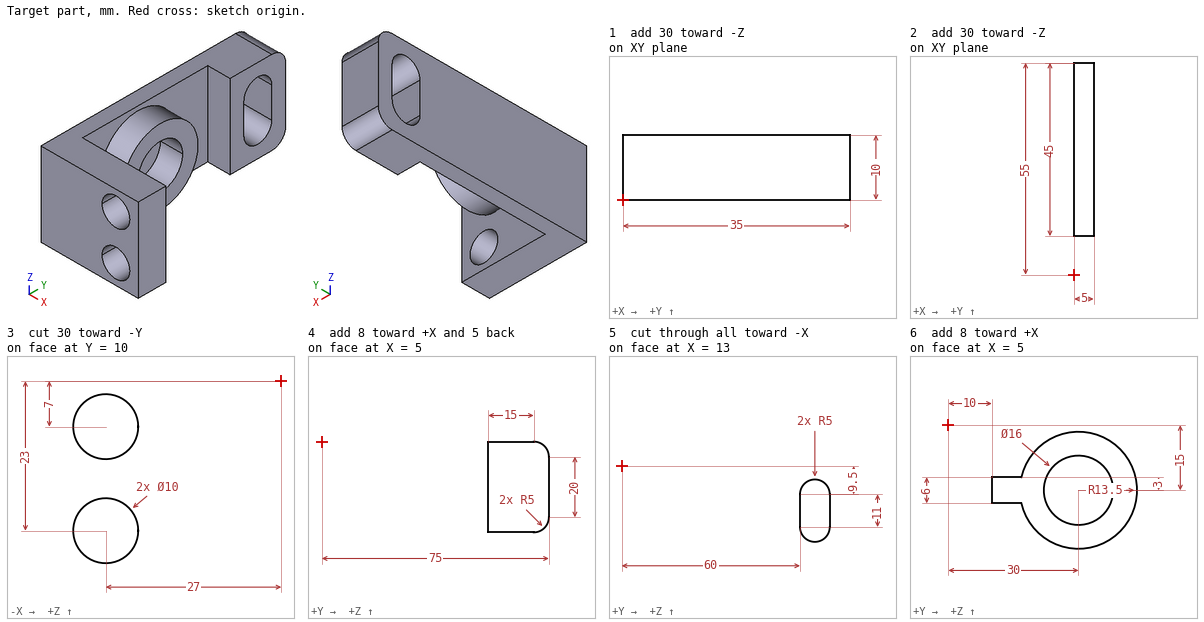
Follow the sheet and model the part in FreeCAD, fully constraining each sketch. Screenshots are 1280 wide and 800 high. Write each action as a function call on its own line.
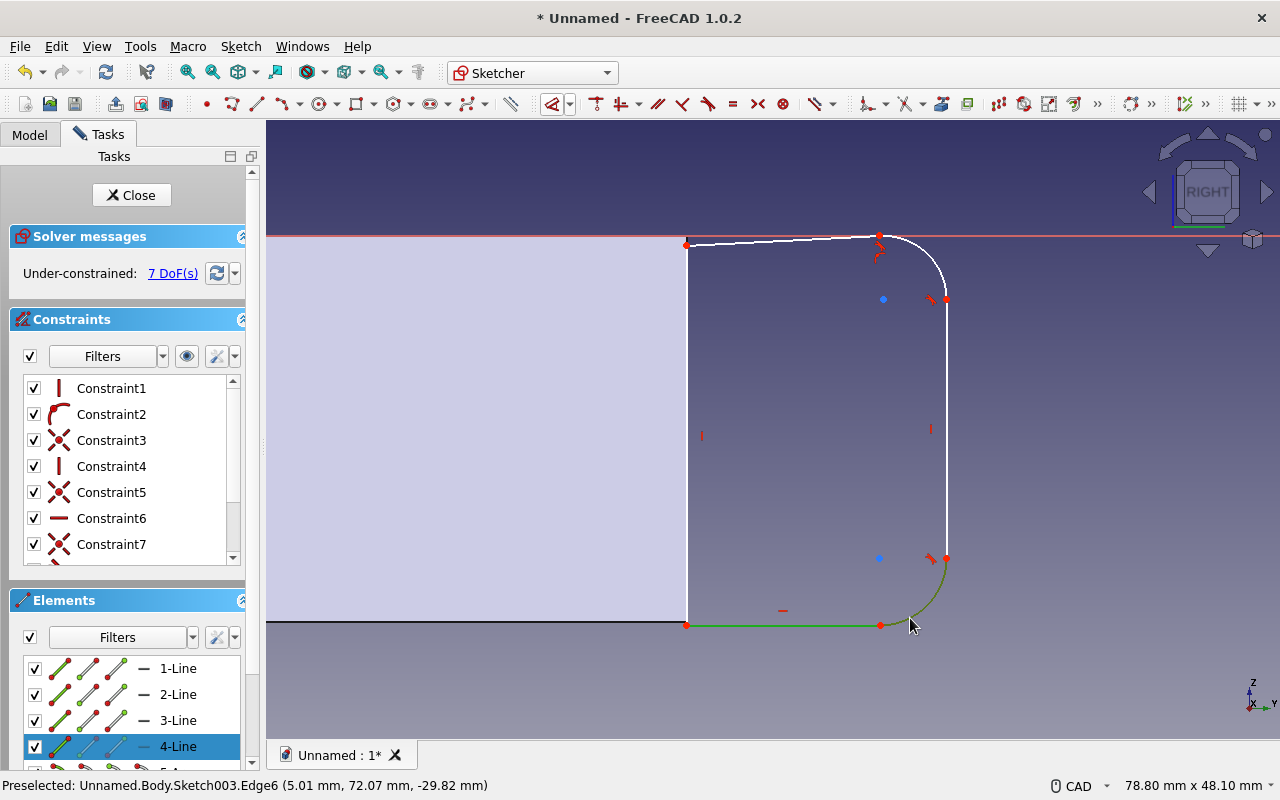
key(t)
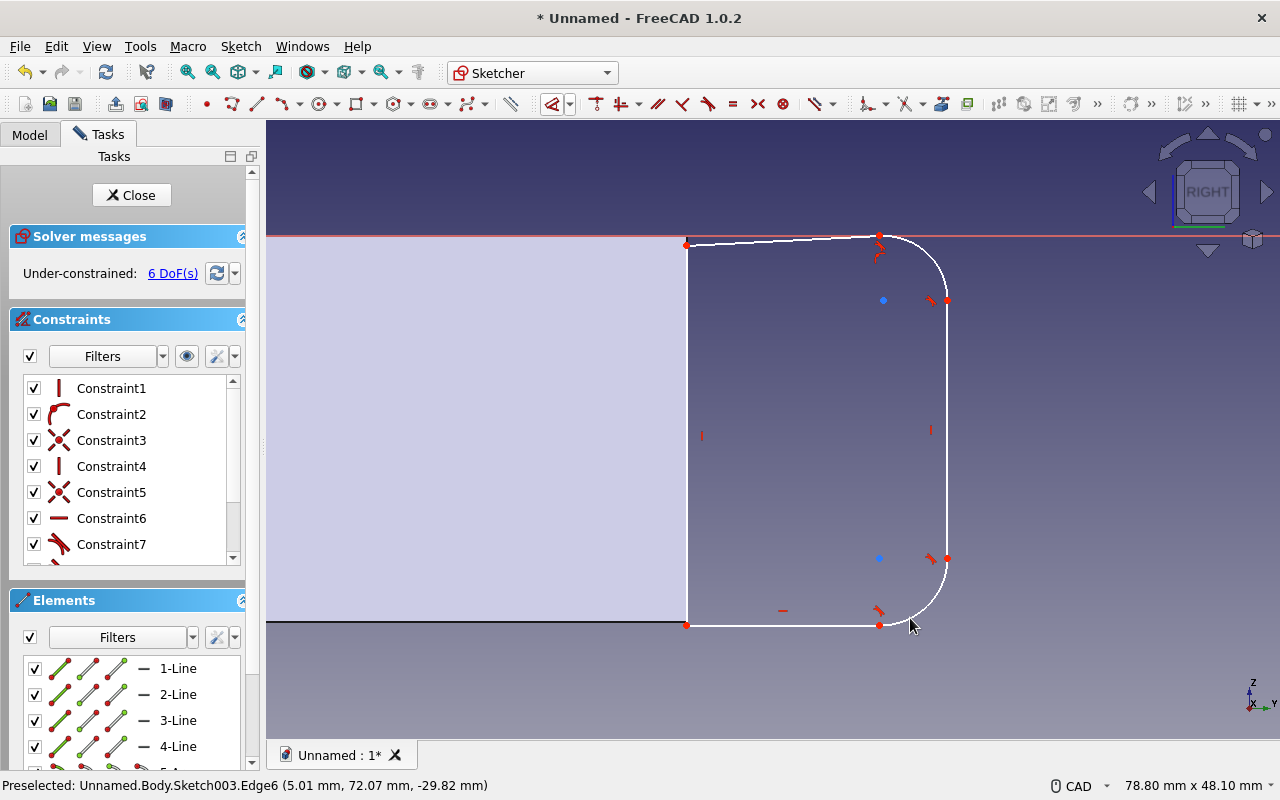
click(822, 239)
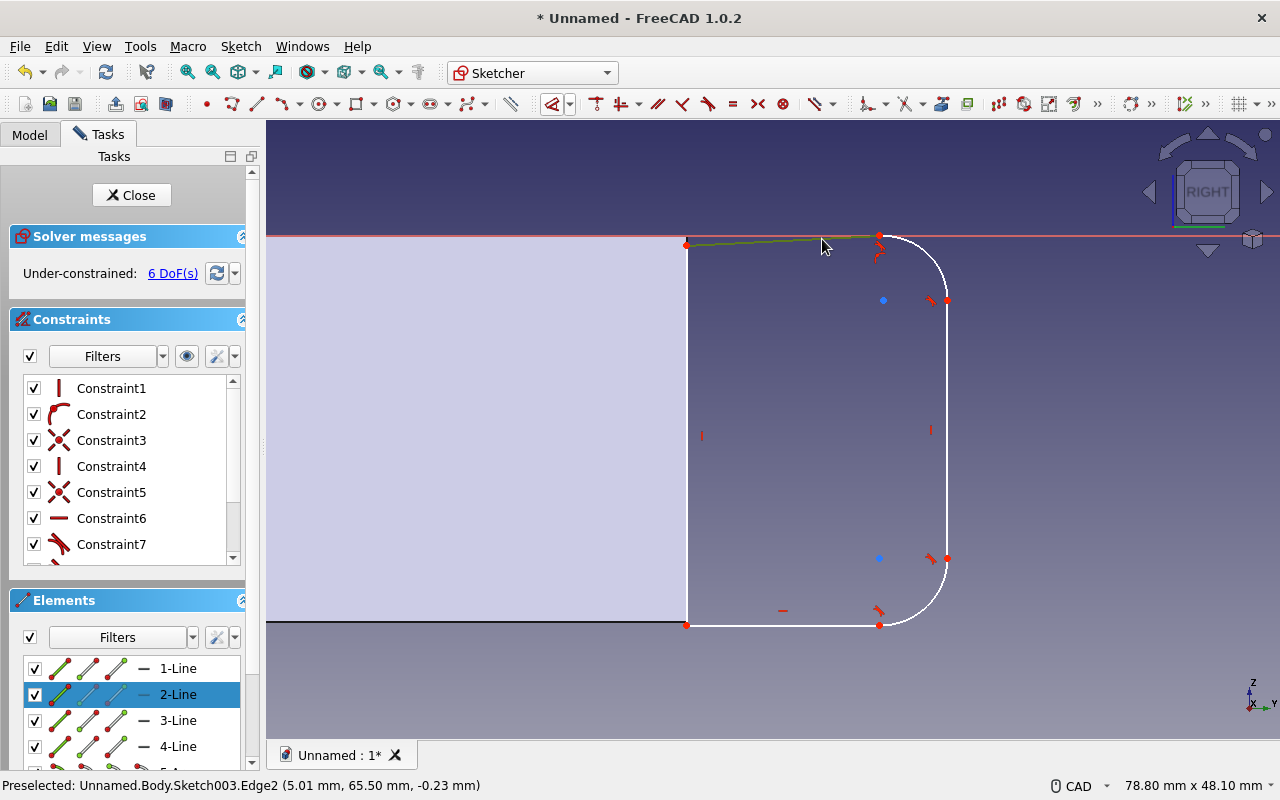
key(h)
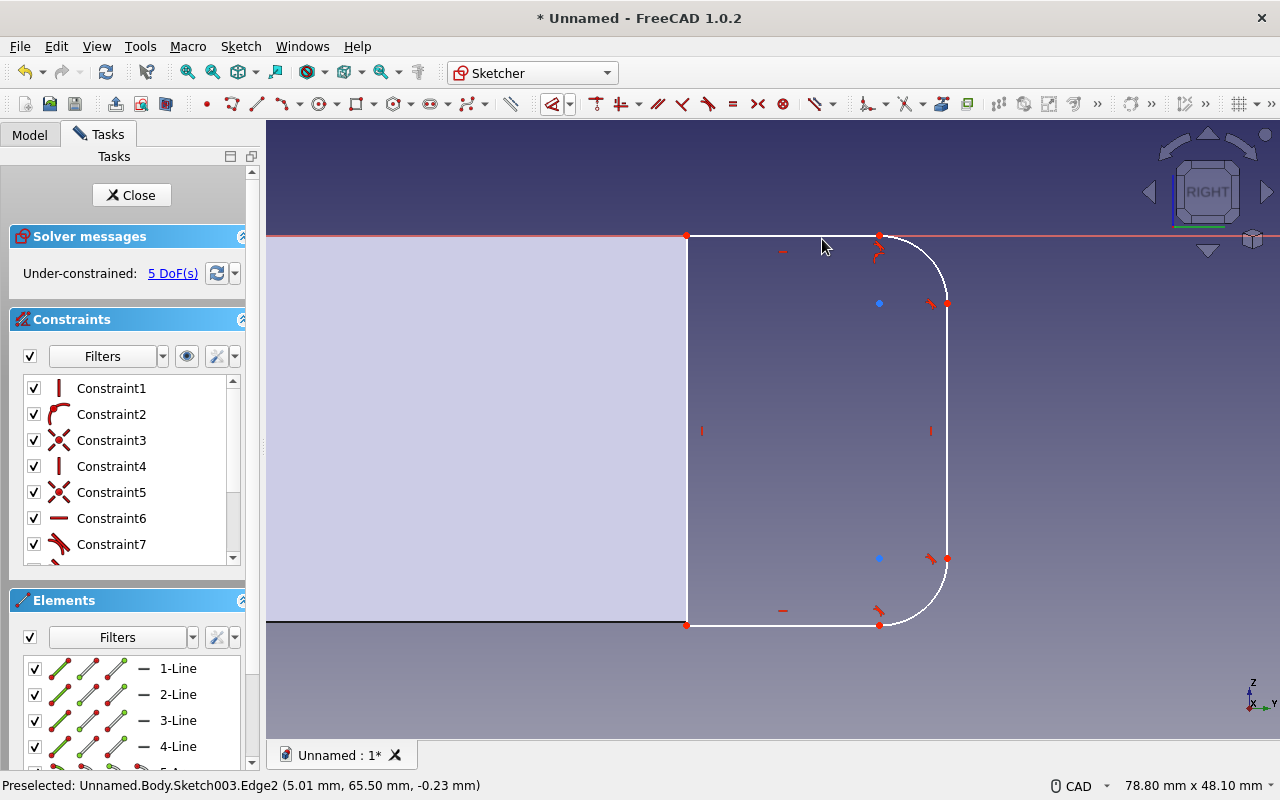
click(940, 273)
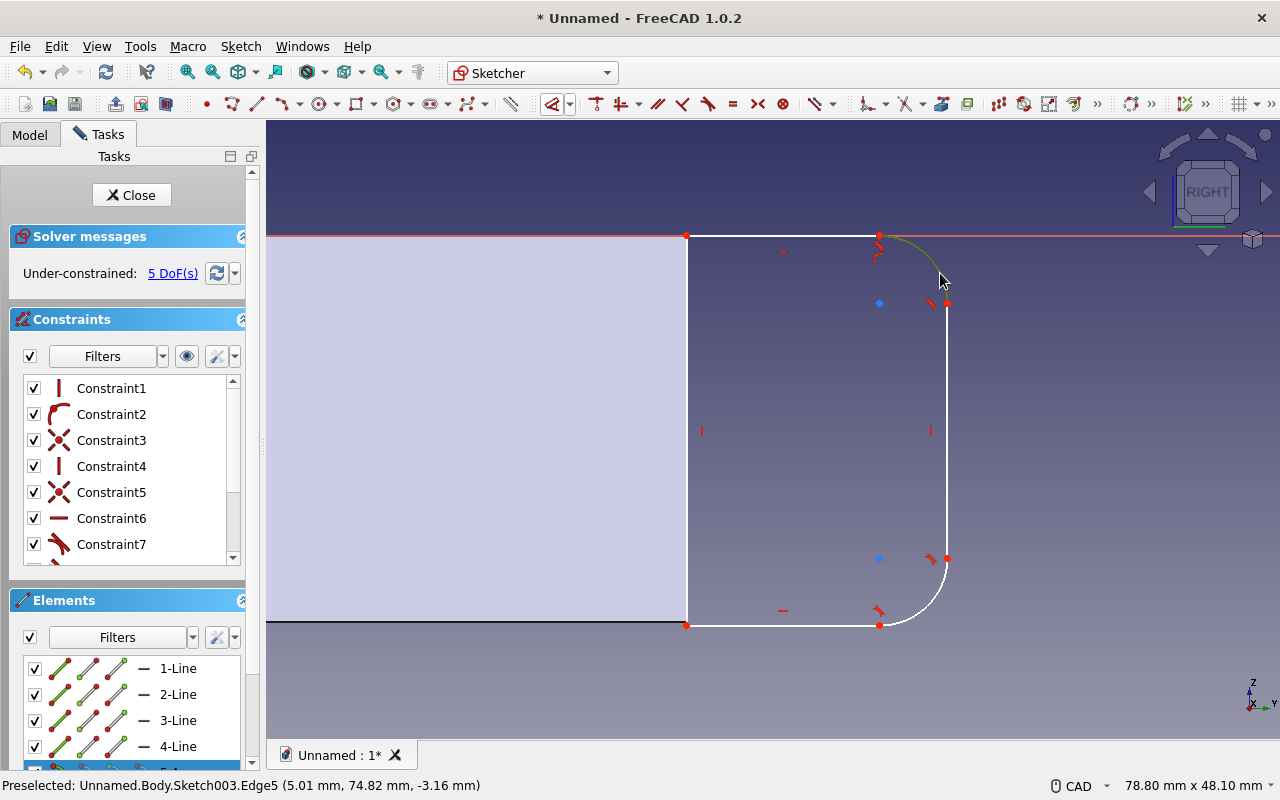
click(911, 618)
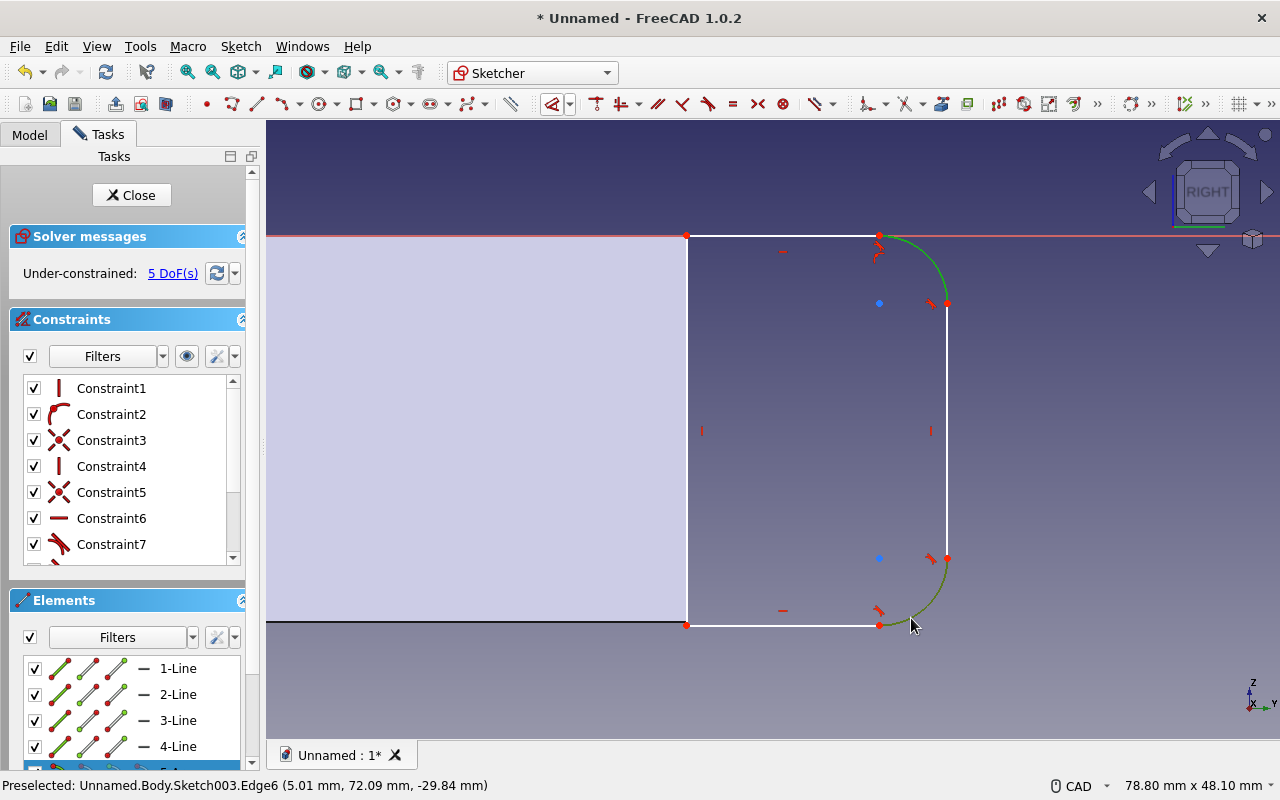
key(e)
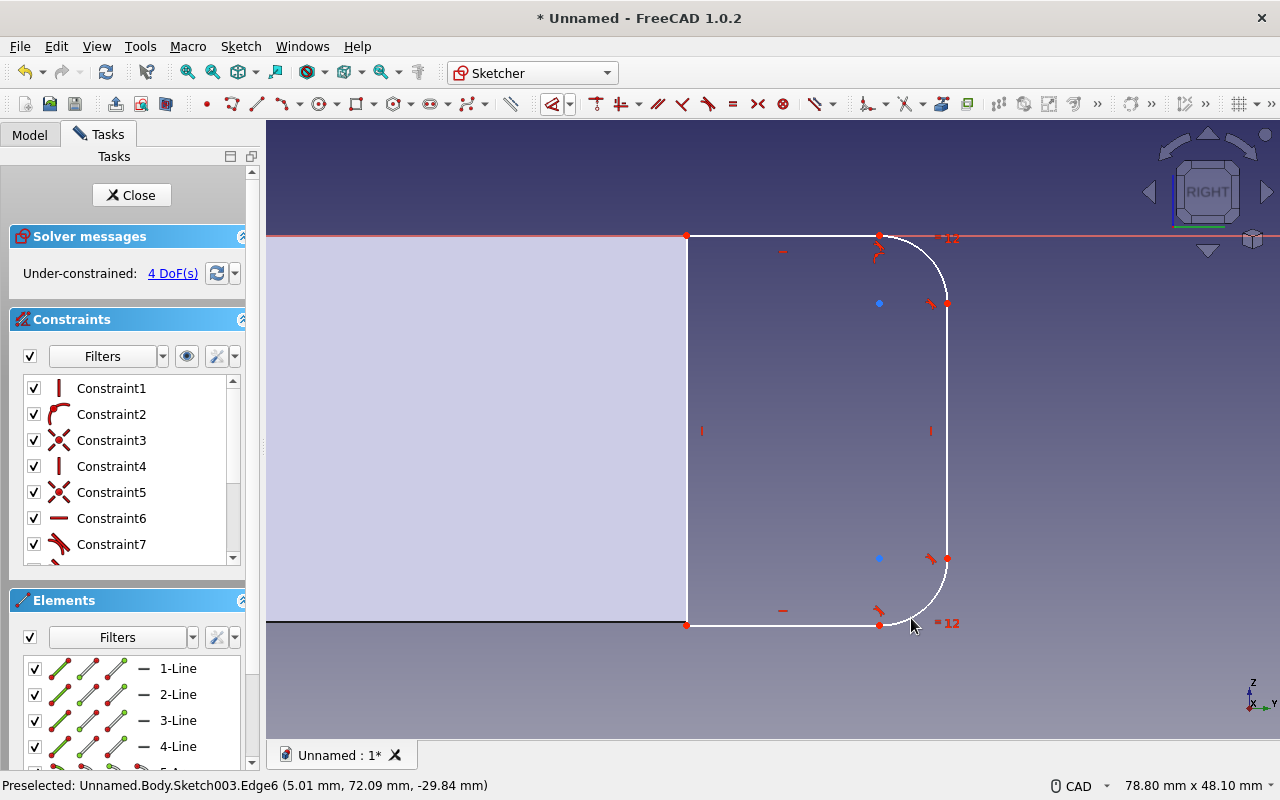
key(d)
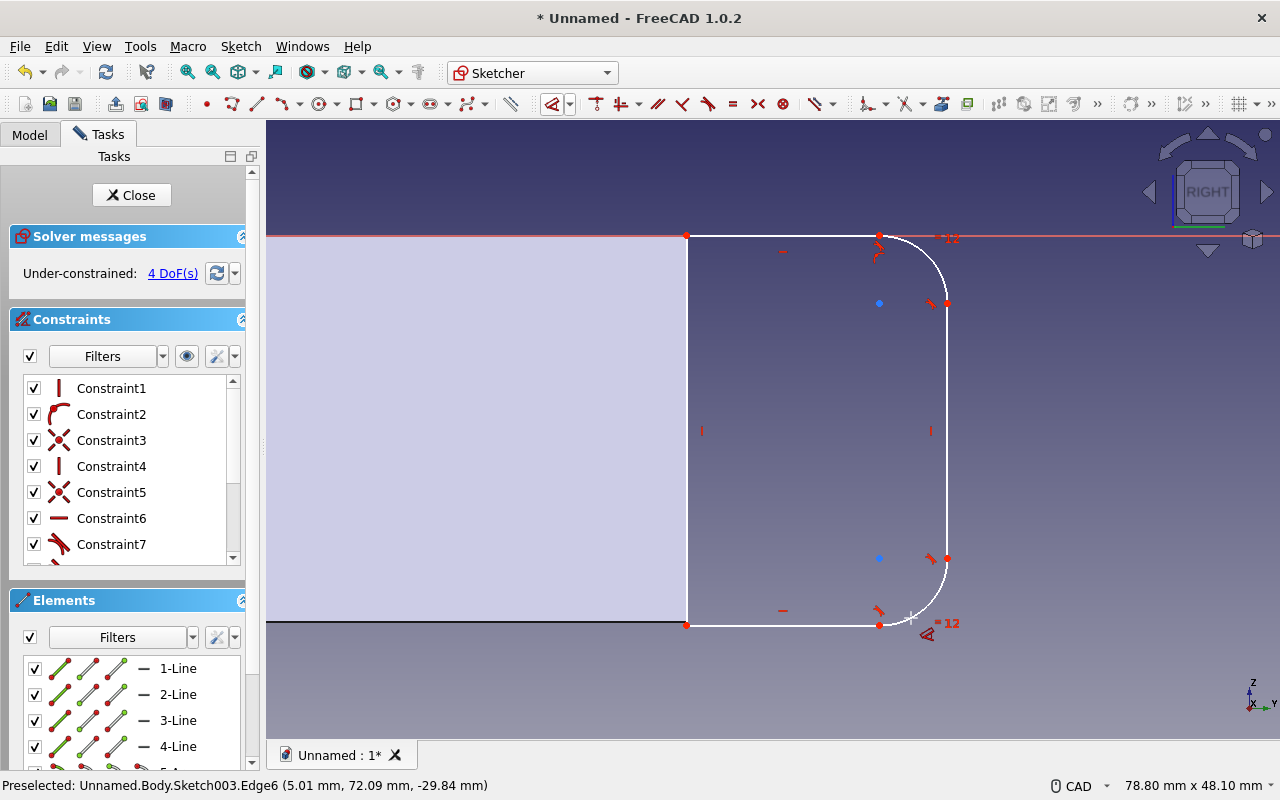
click(940, 273)
click(969, 259)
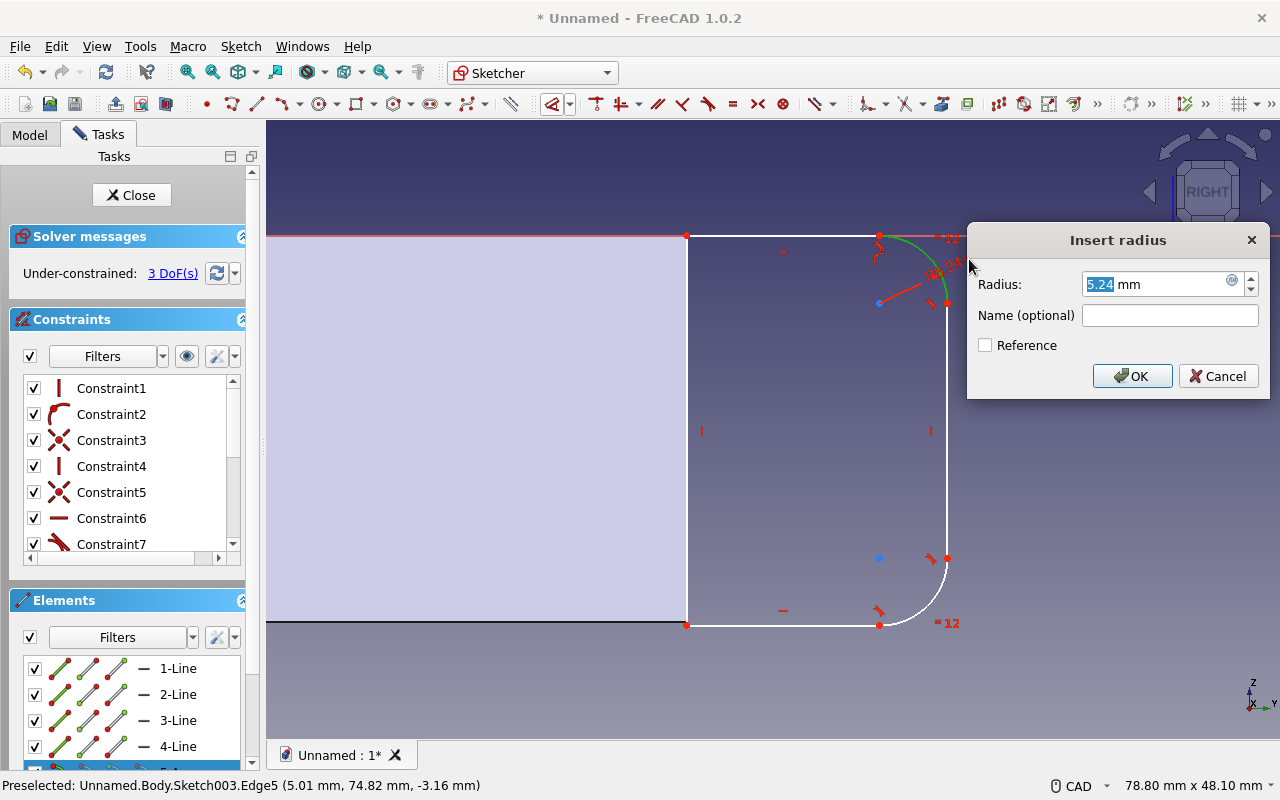
text(5)
key(Return)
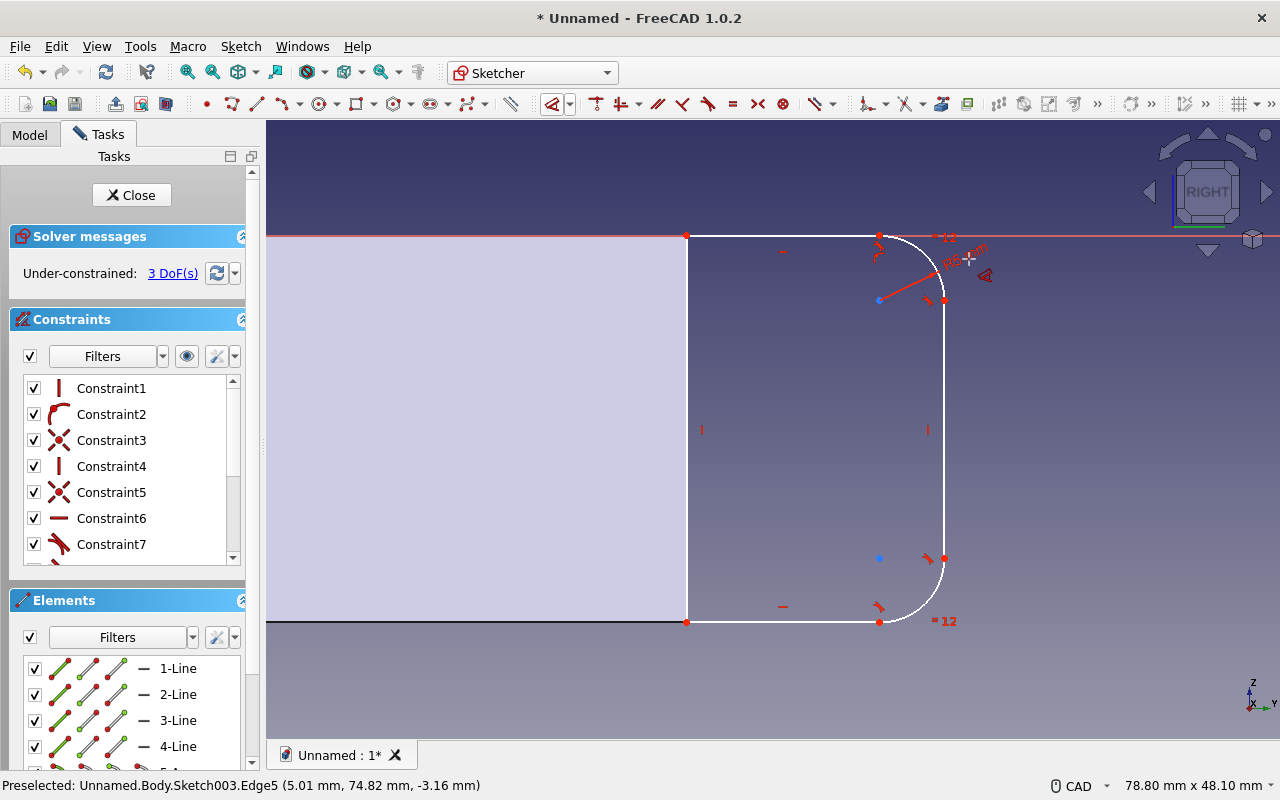
click(944, 481)
click(978, 429)